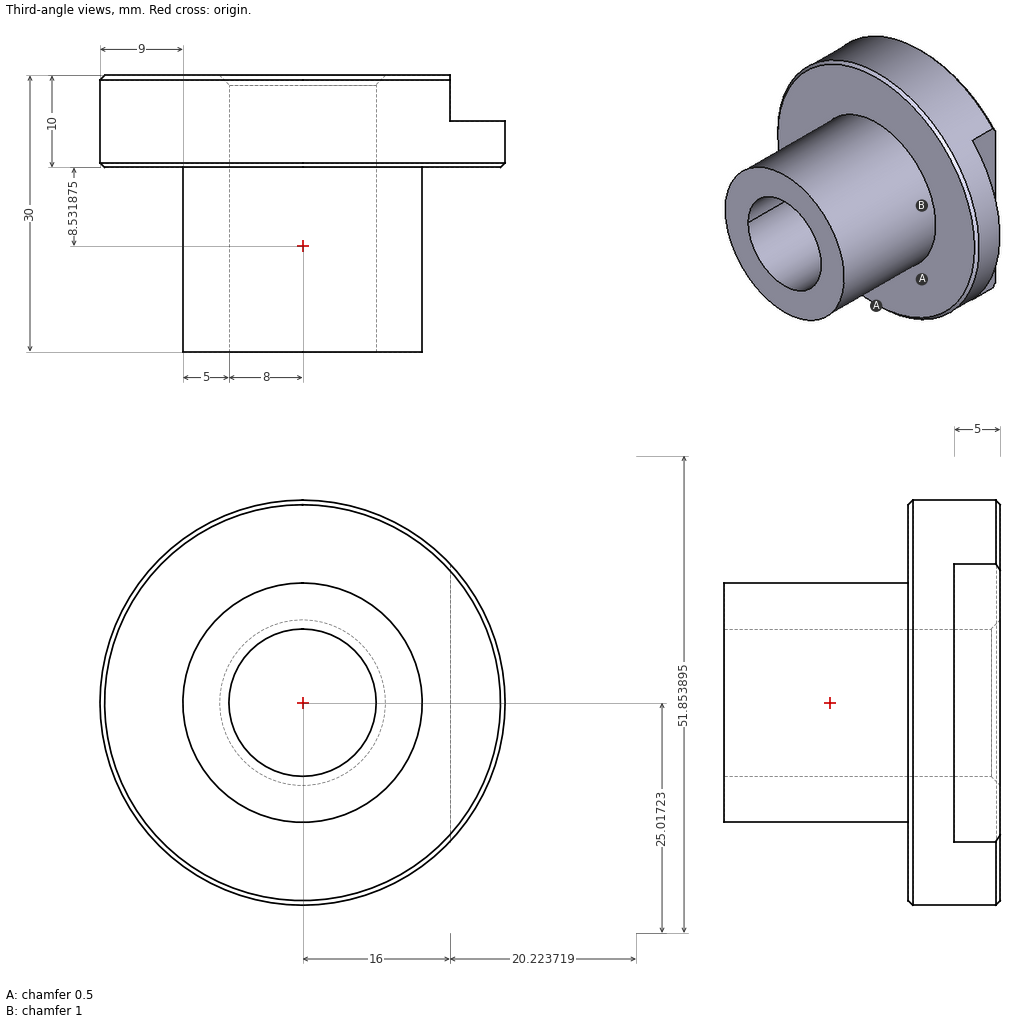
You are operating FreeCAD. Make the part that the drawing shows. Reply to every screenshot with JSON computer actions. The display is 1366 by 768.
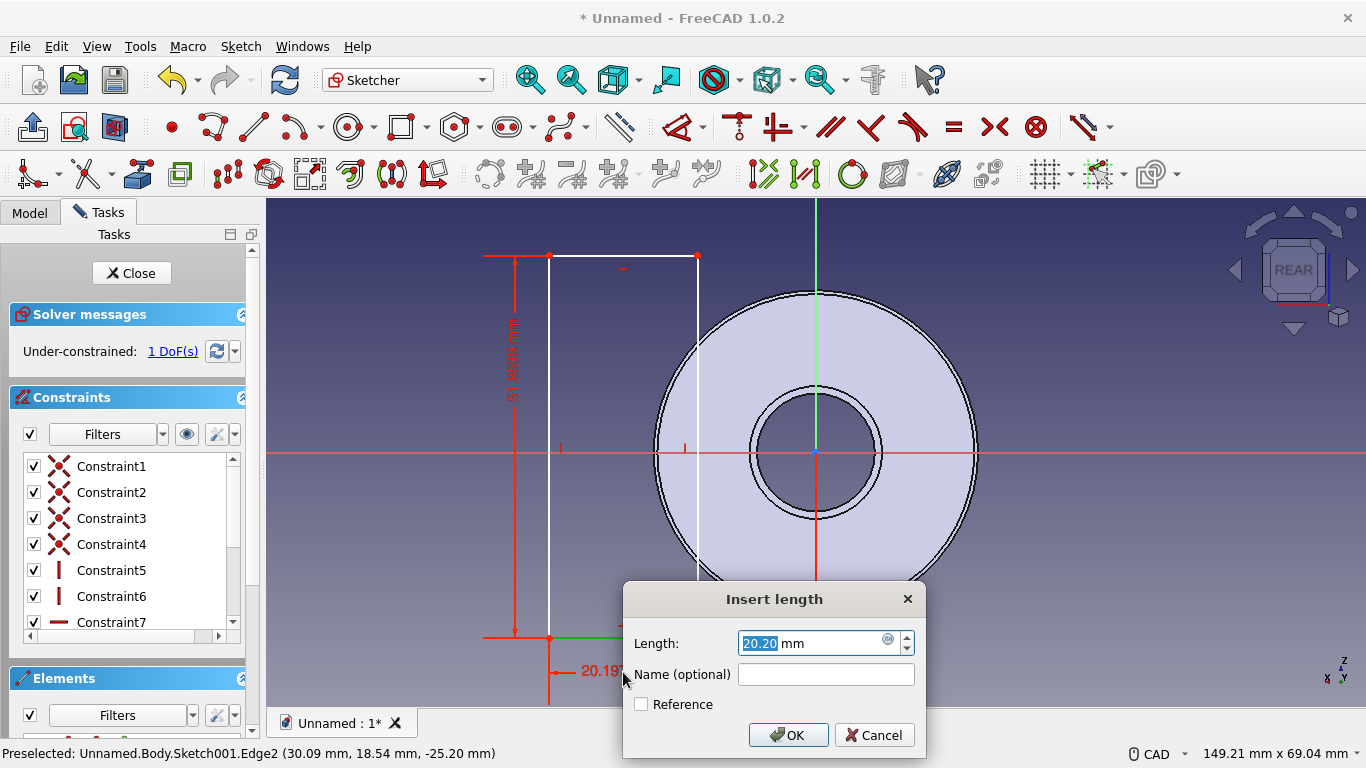
{"action": "type", "text": "20.223719"}
{"action": "key", "text": "Return"}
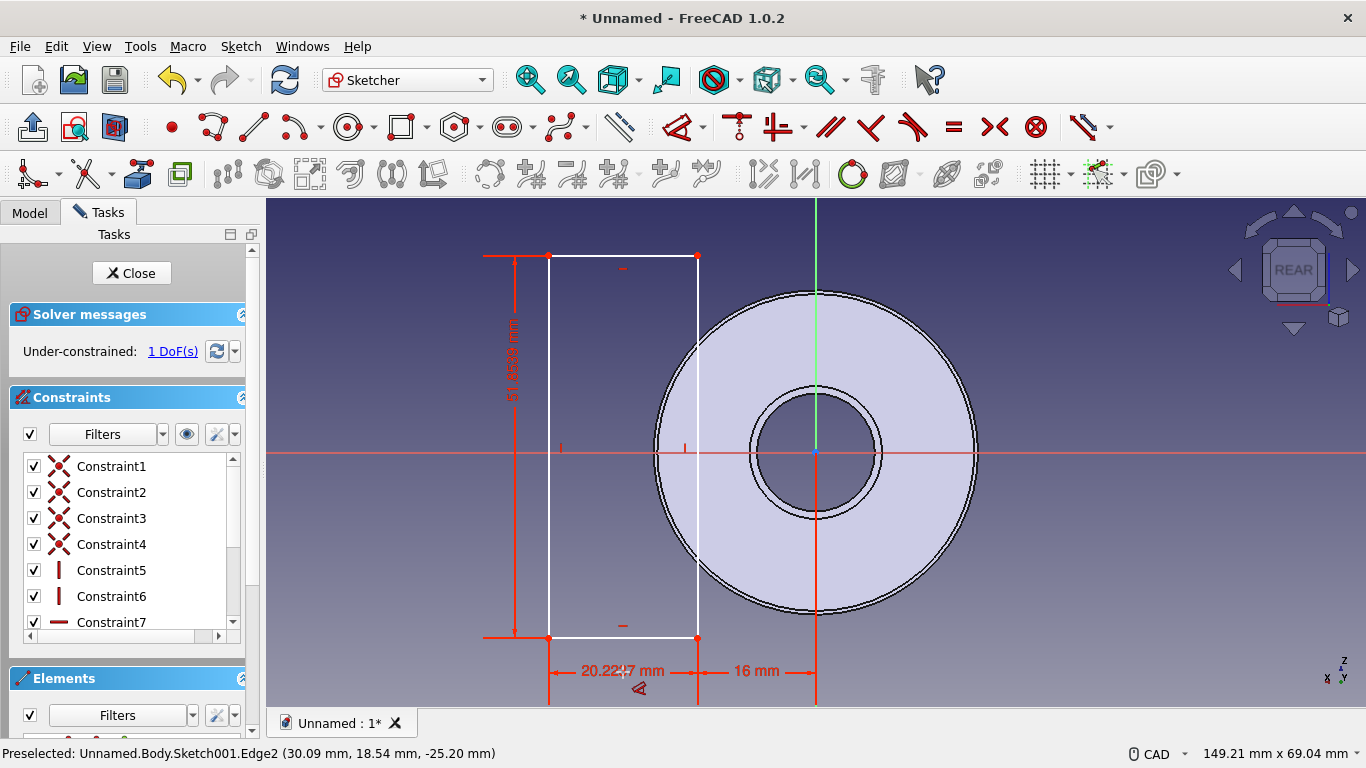
{"action": "left_click", "coordinate": [549, 638]}
{"action": "left_click", "coordinate": [515, 545]}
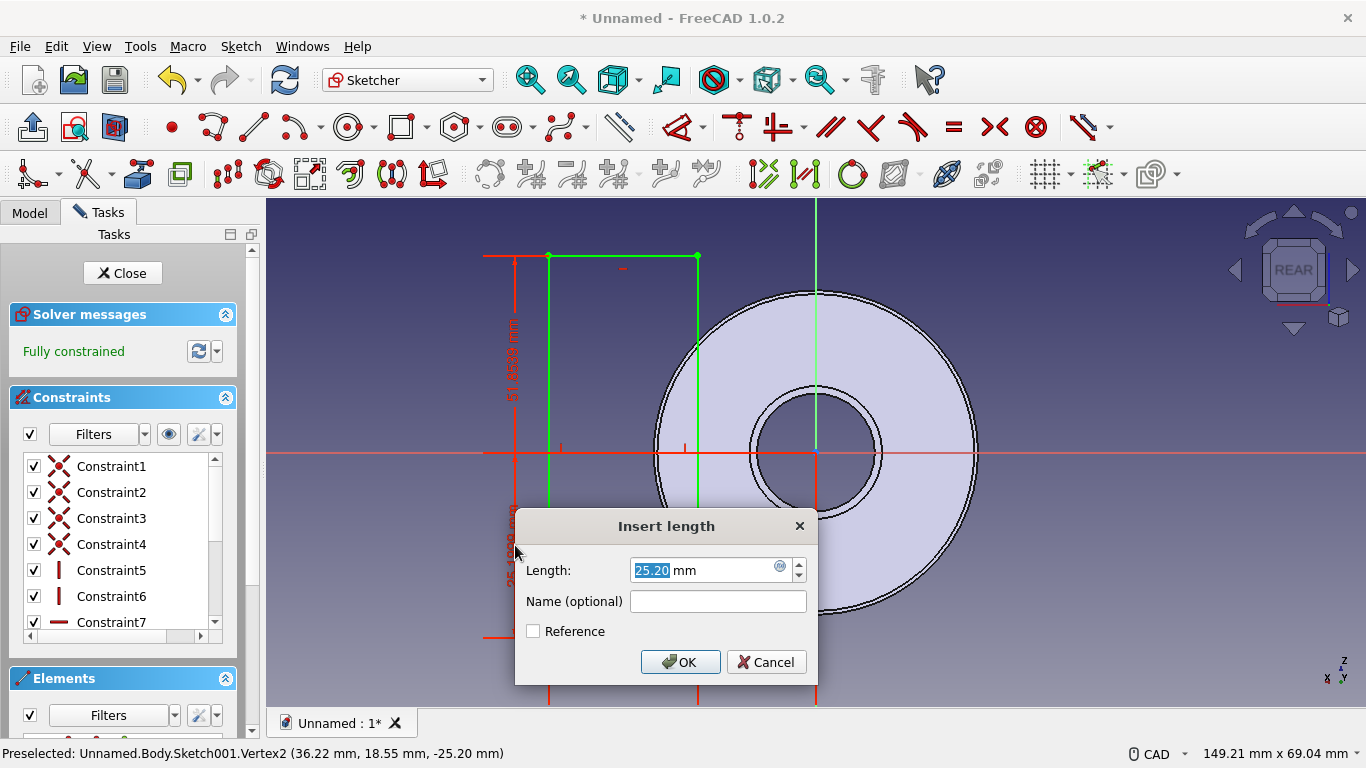
{"action": "type", "text": "25.01723"}
{"action": "key", "text": "Return"}
{"action": "key", "text": "Escape"}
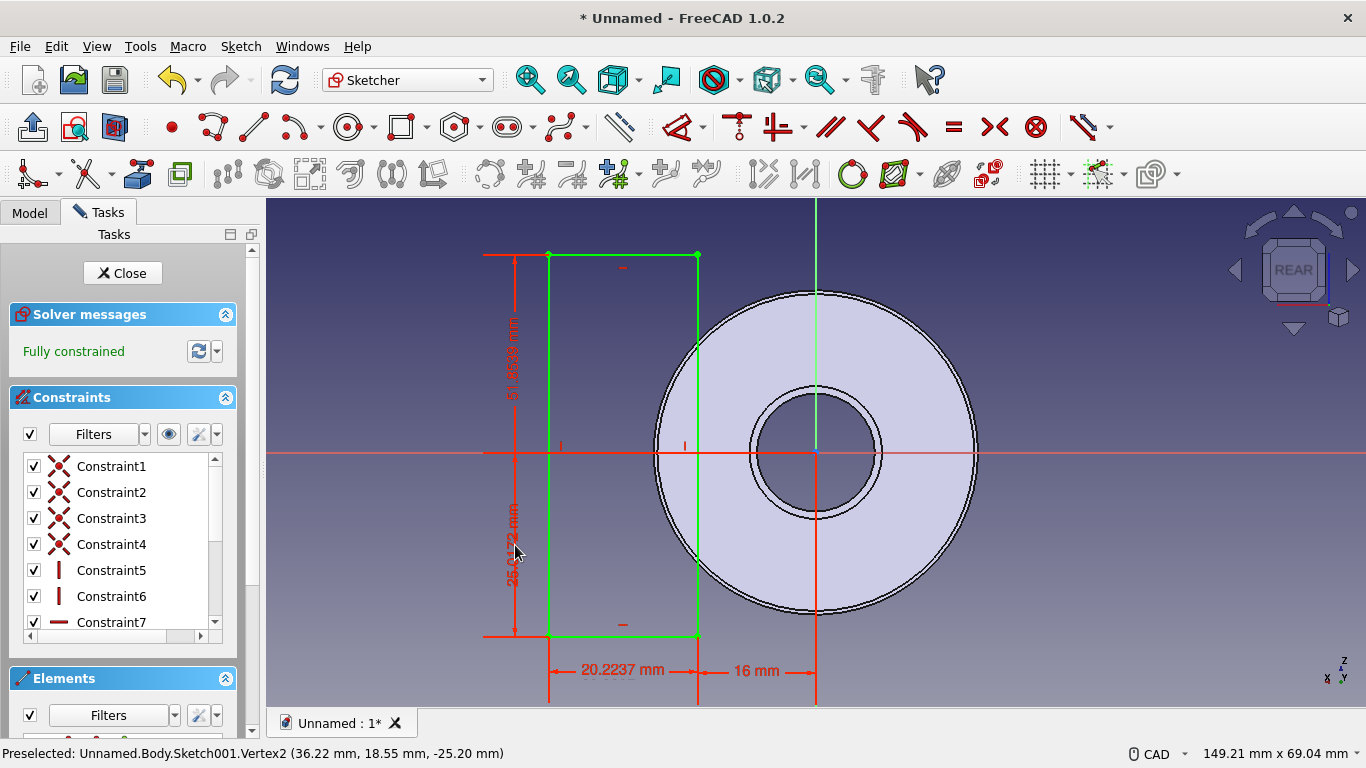
{"action": "left_click", "coordinate": [123, 273]}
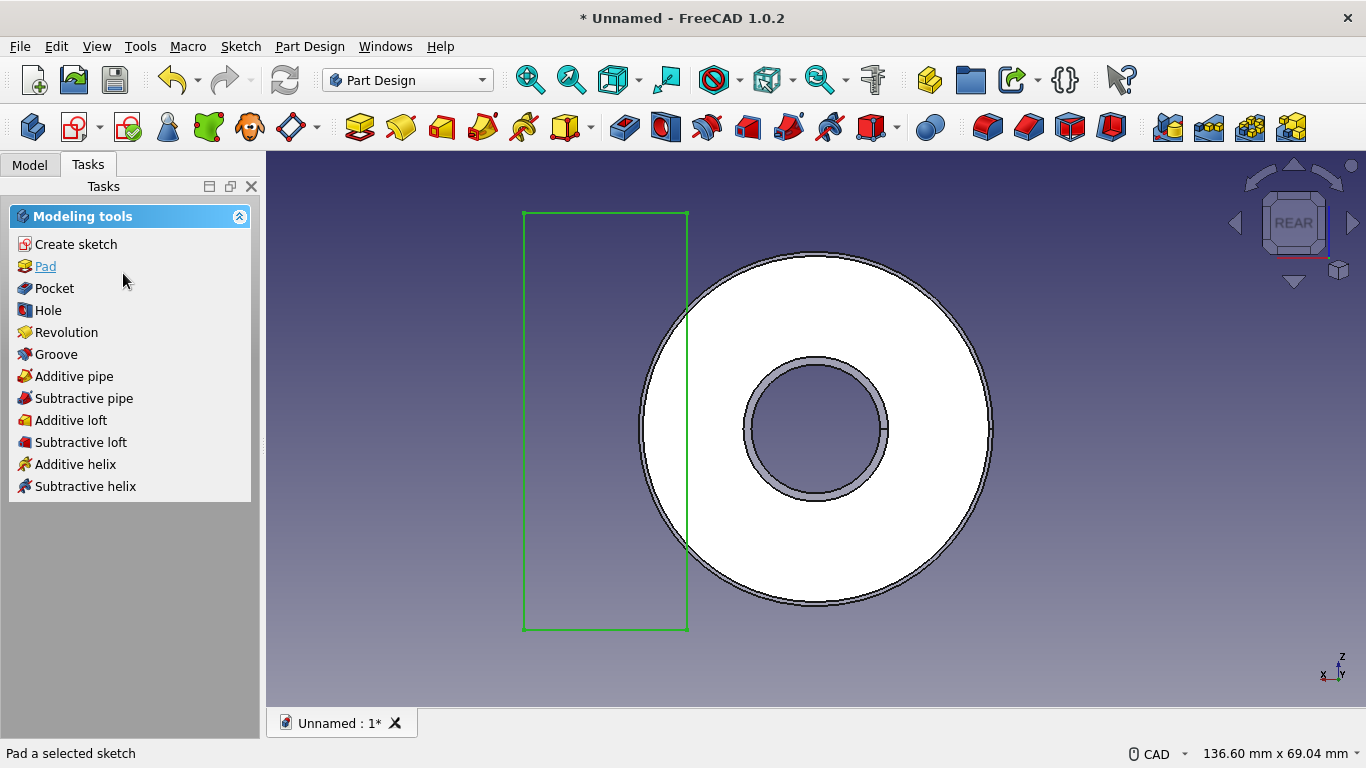
{"action": "left_click", "coordinate": [625, 128]}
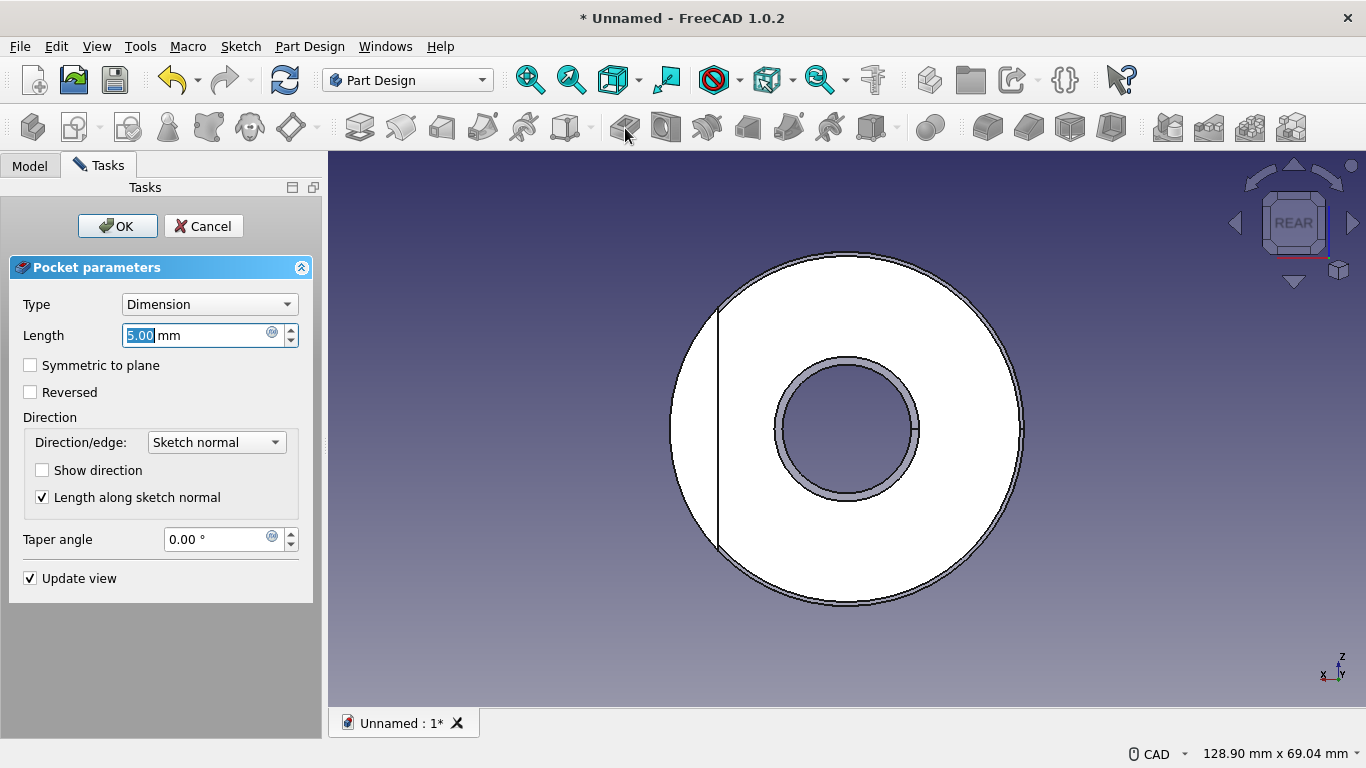
{"action": "type", "text": "5"}
{"action": "key", "text": "Tab"}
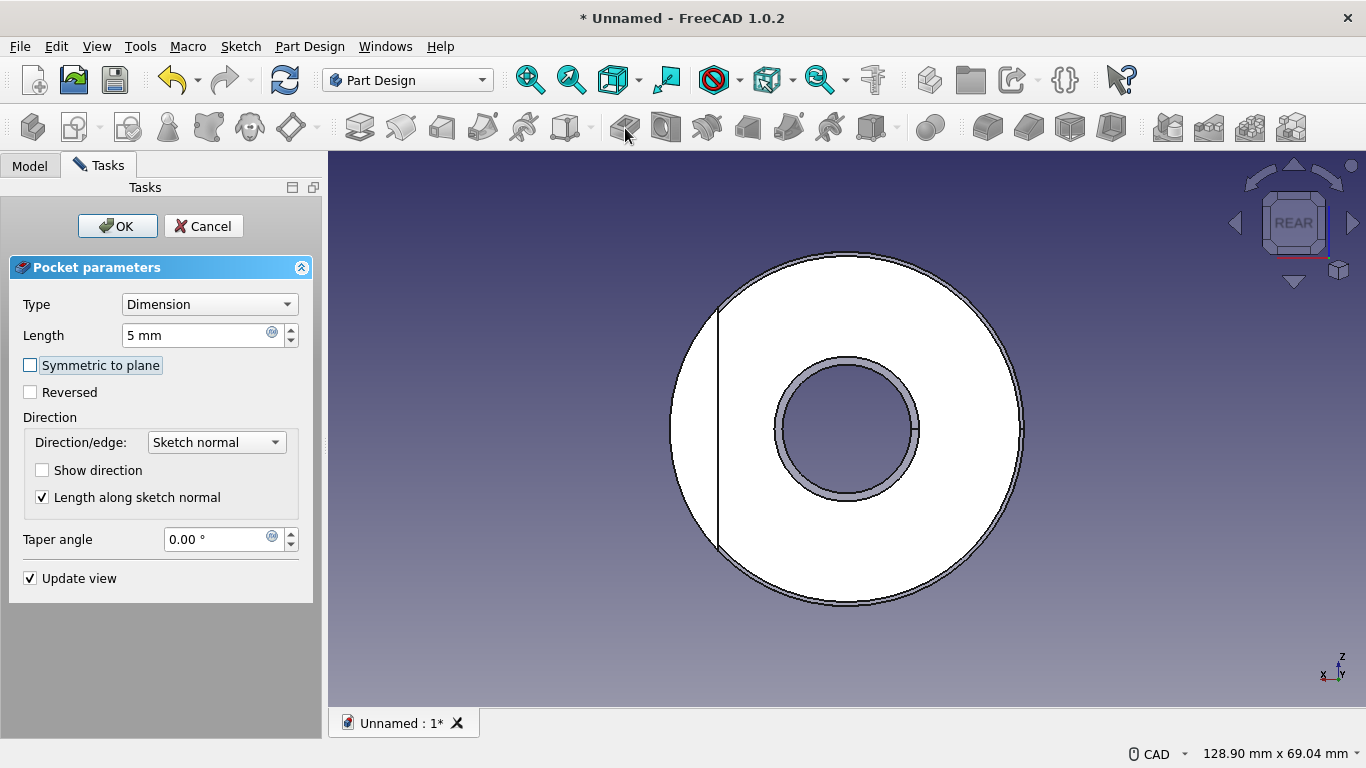
{"action": "left_click", "coordinate": [118, 226]}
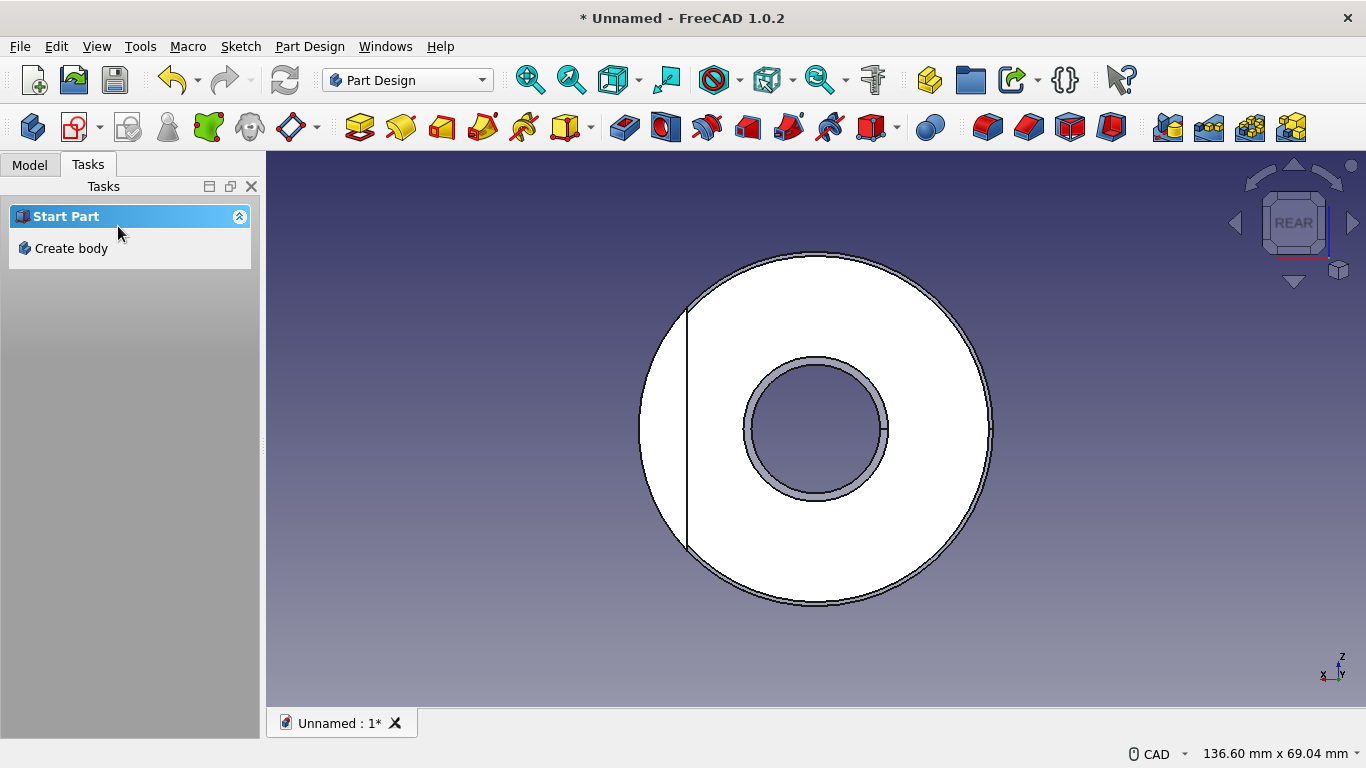
{"action": "key", "text": "0"}